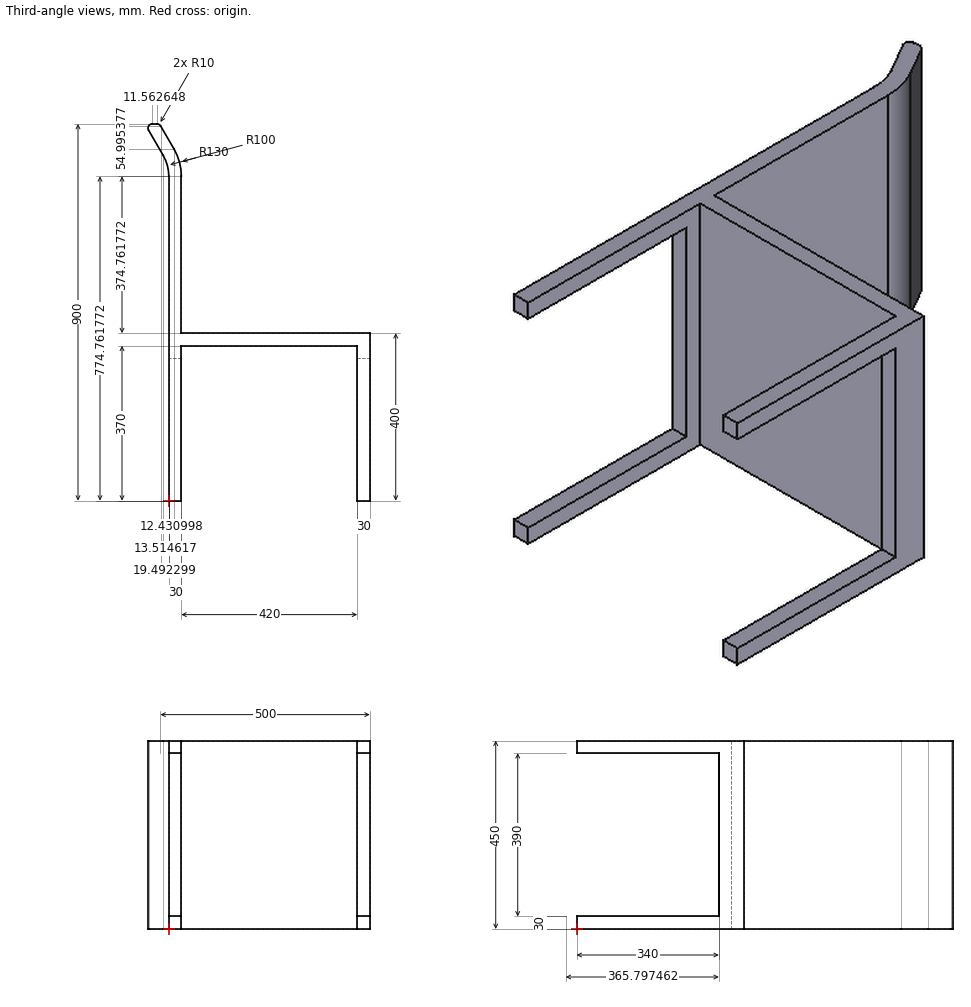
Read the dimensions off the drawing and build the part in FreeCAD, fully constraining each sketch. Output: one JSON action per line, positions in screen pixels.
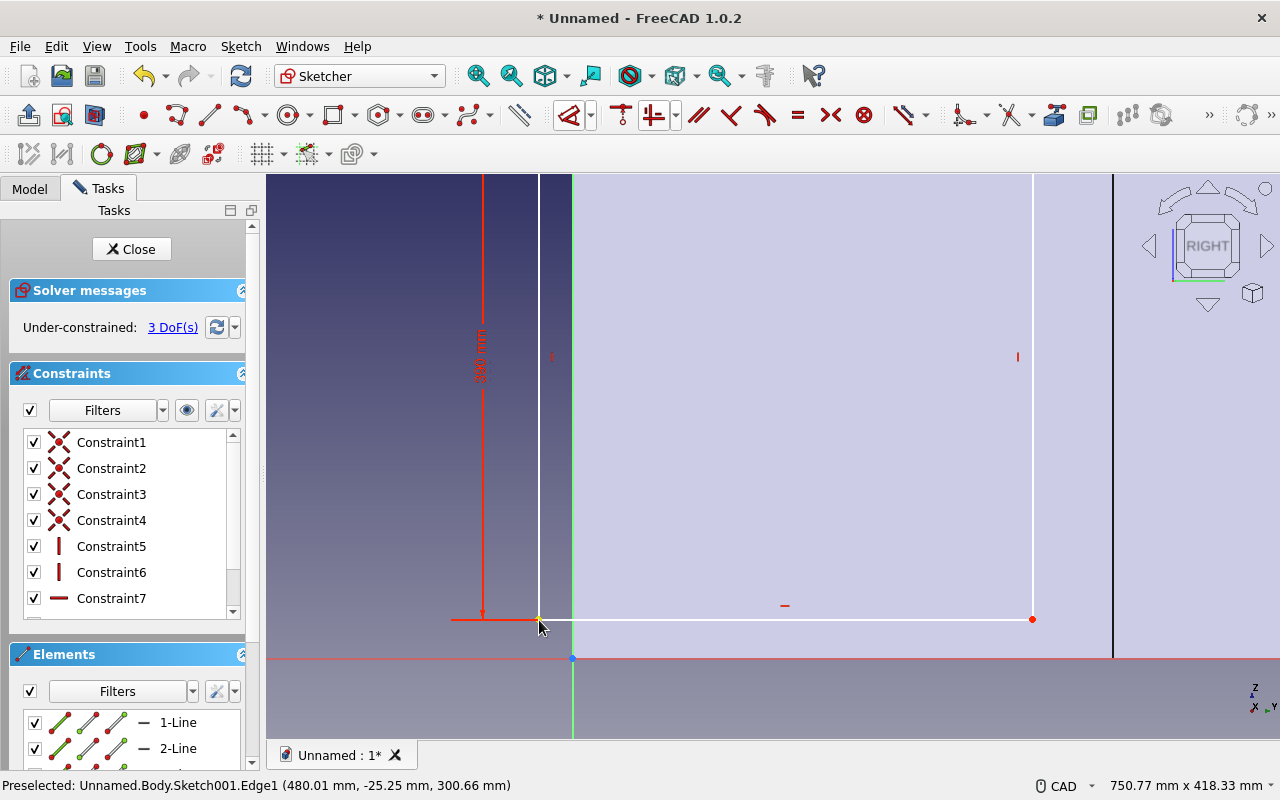
{"action": "left_click", "coordinate": [539, 620]}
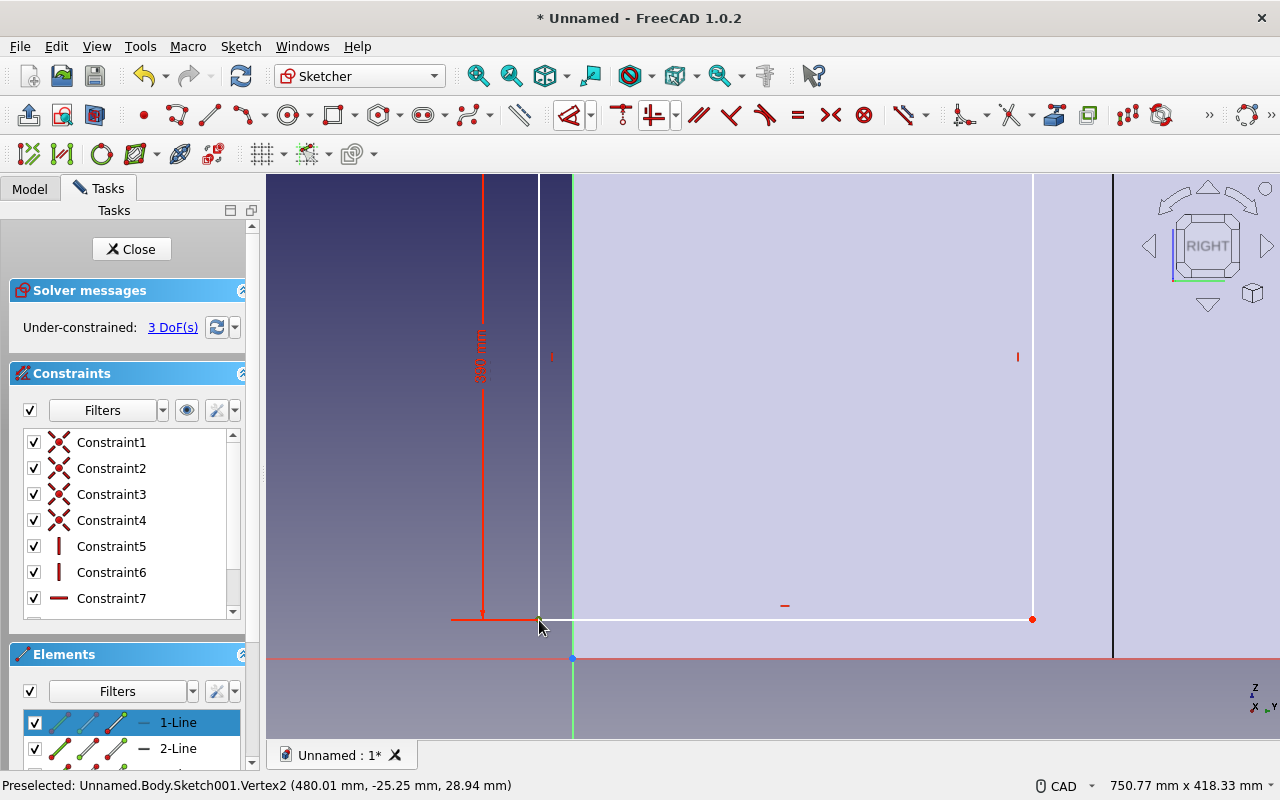
{"action": "left_click", "coordinate": [590, 116]}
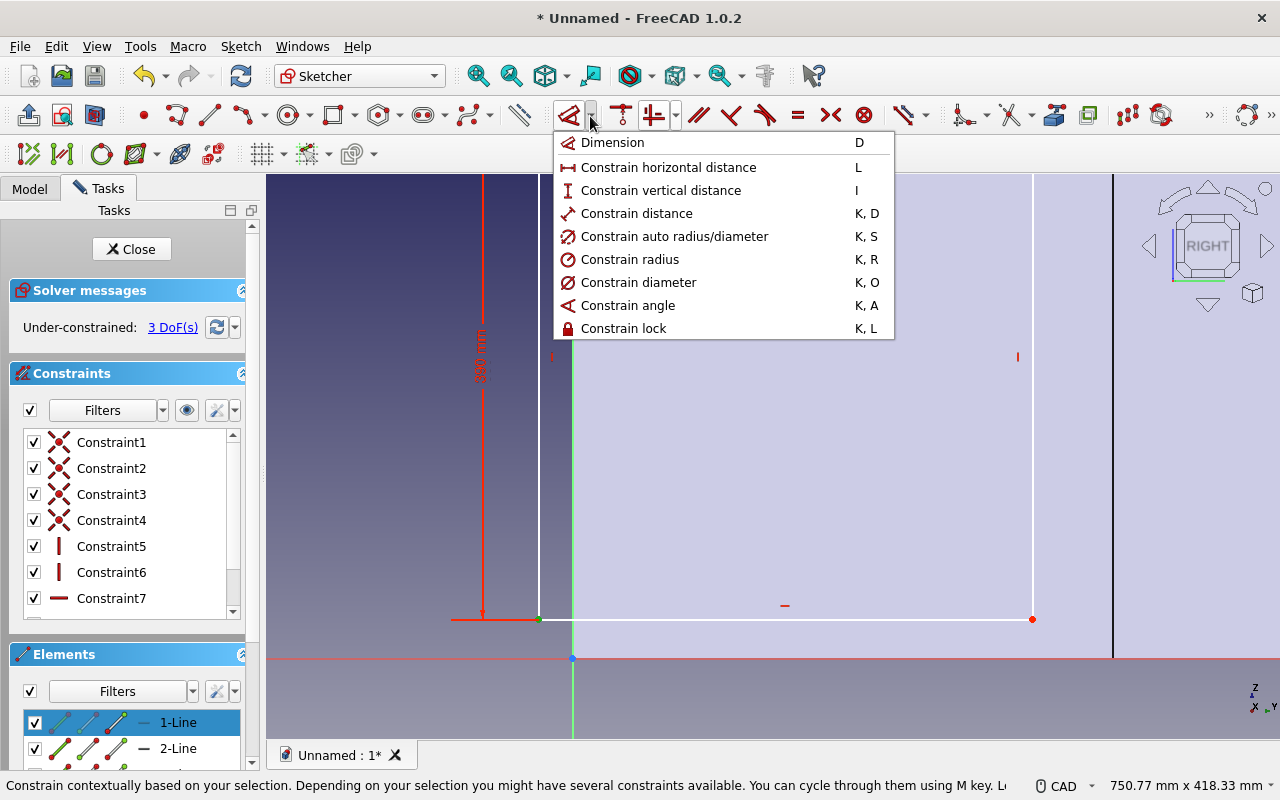
{"action": "left_click", "coordinate": [724, 190]}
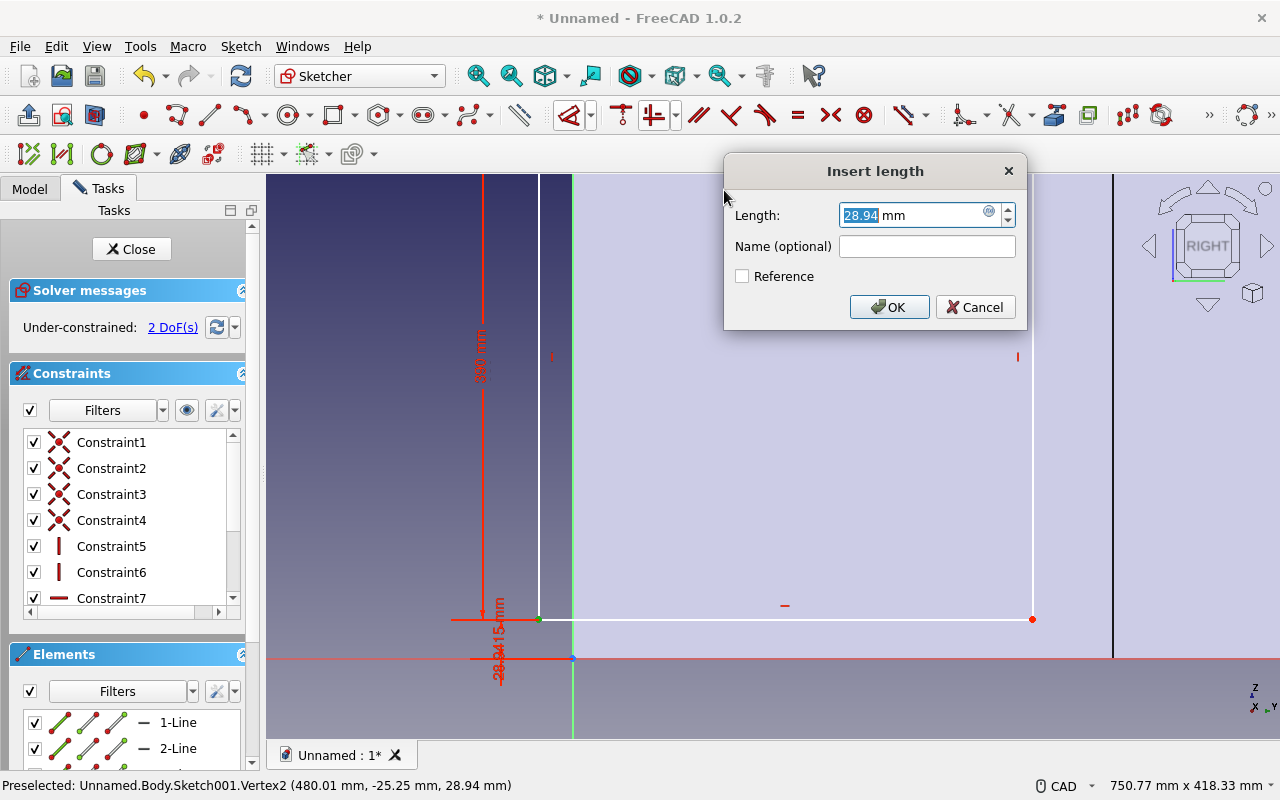
{"action": "type", "text": "30"}
{"action": "key", "text": "Return"}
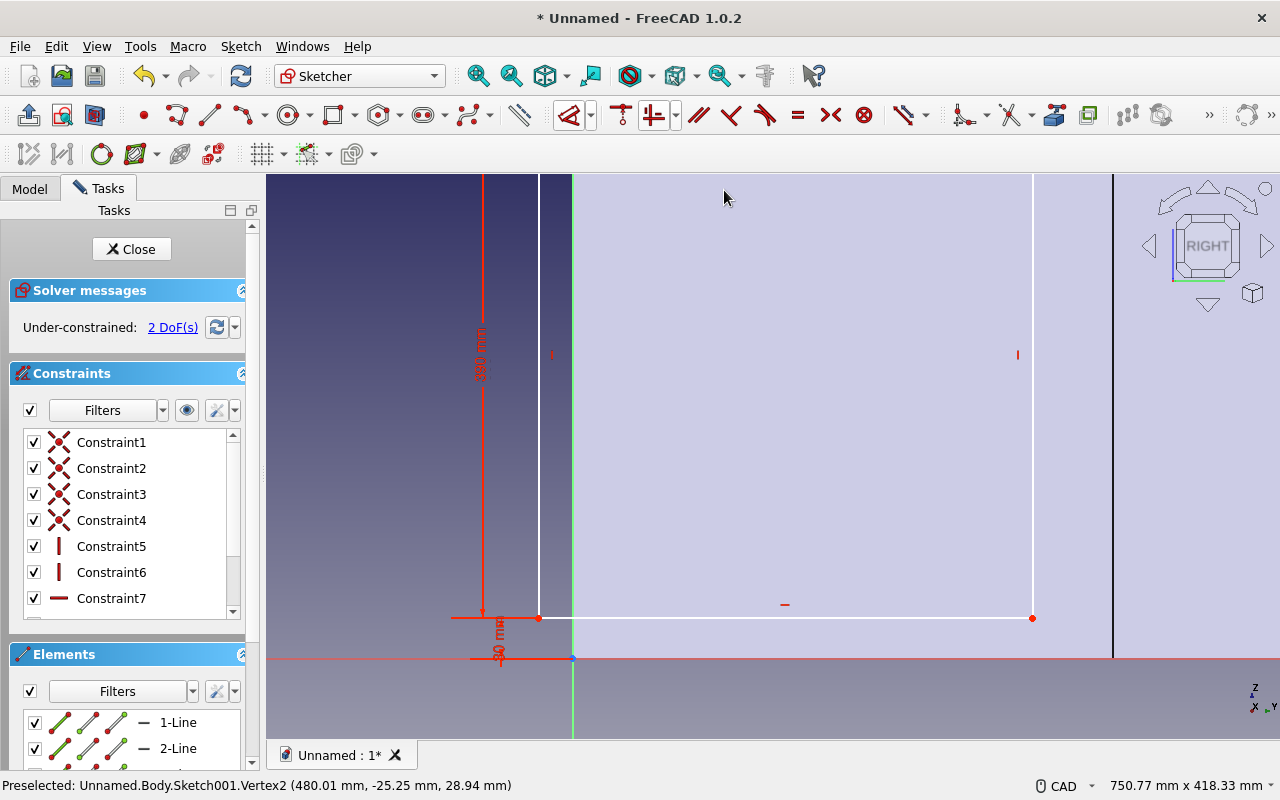
{"action": "left_click", "coordinate": [1033, 618]}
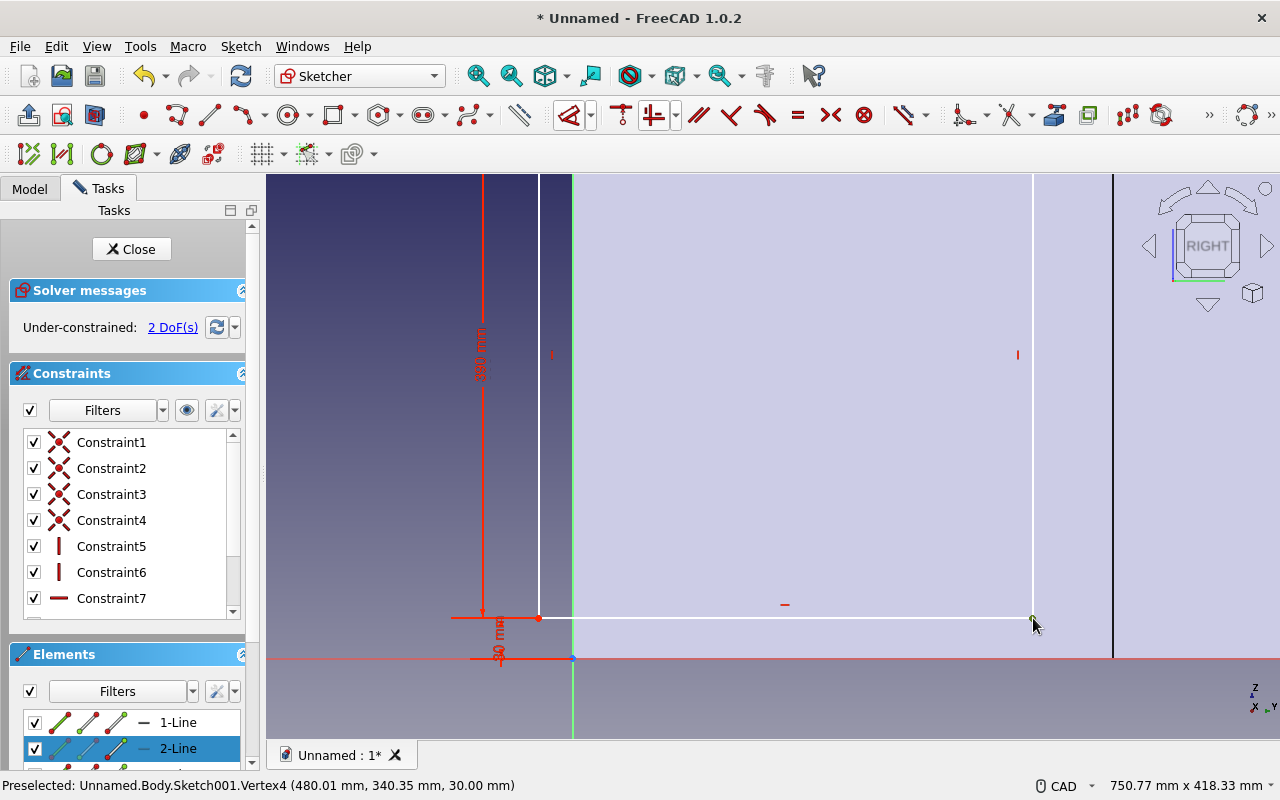
{"action": "left_click", "coordinate": [590, 116]}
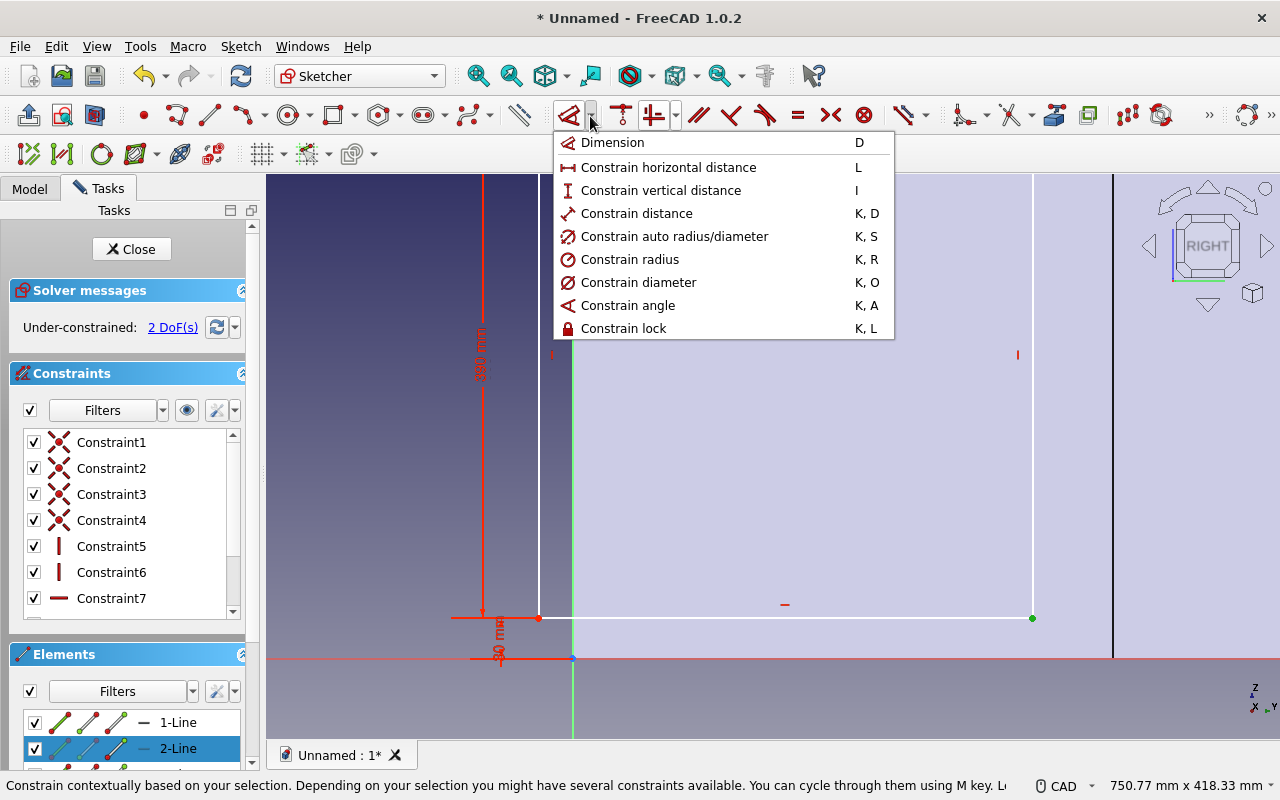
{"action": "left_click", "coordinate": [724, 168]}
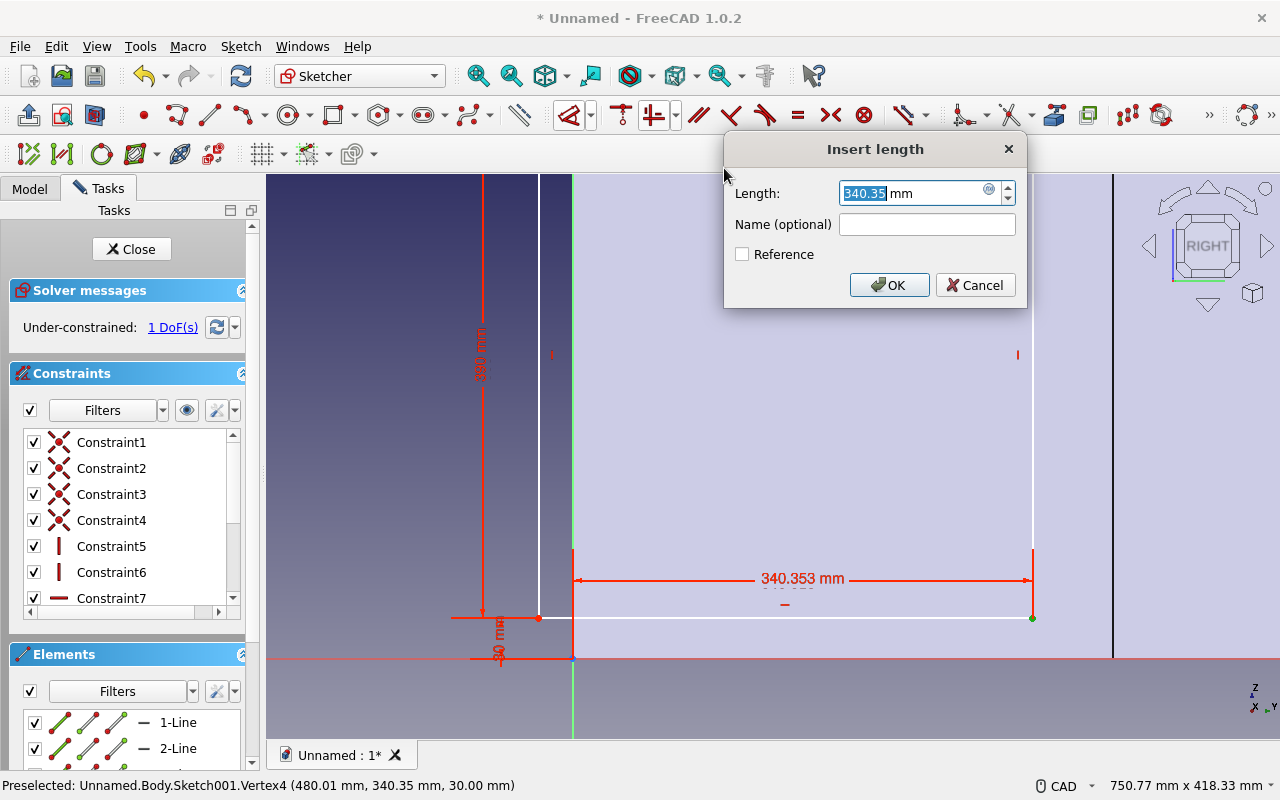
{"action": "type", "text": "340"}
{"action": "key", "text": "Return"}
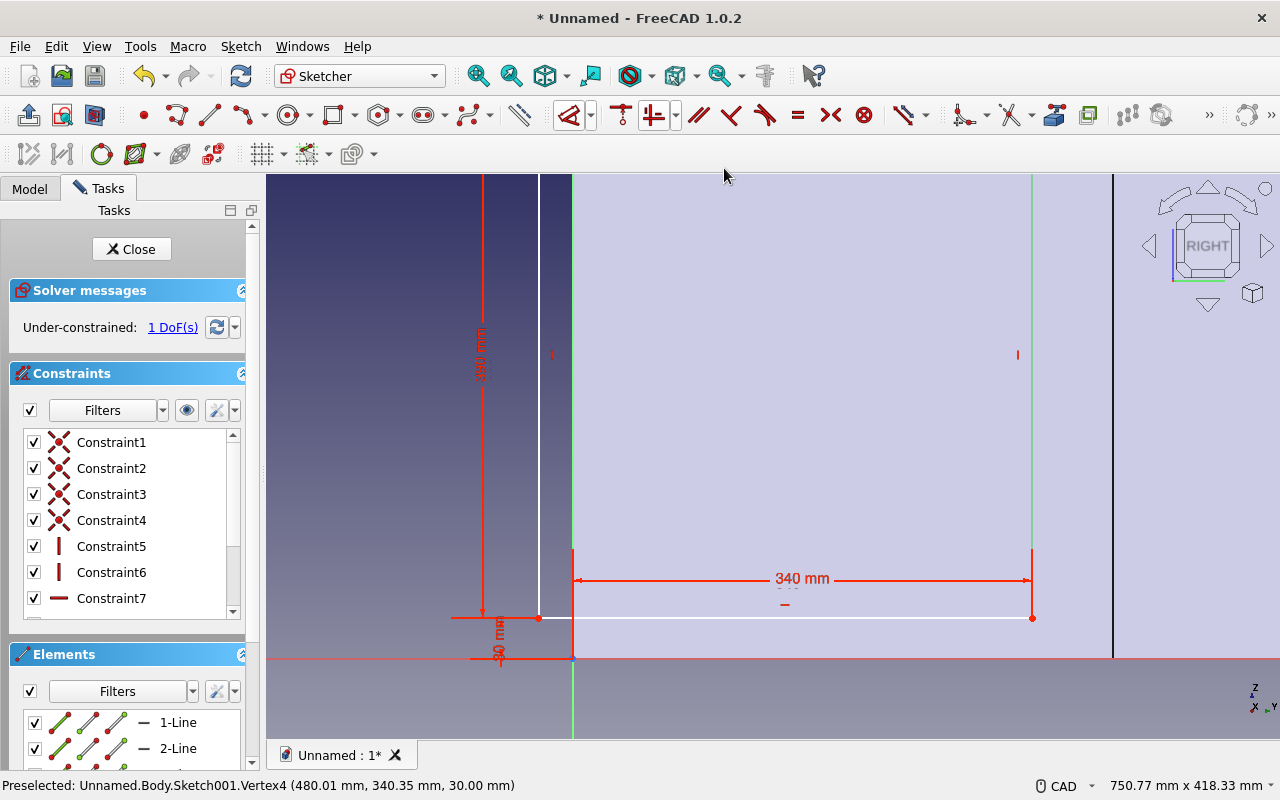
{"action": "left_click", "coordinate": [687, 618]}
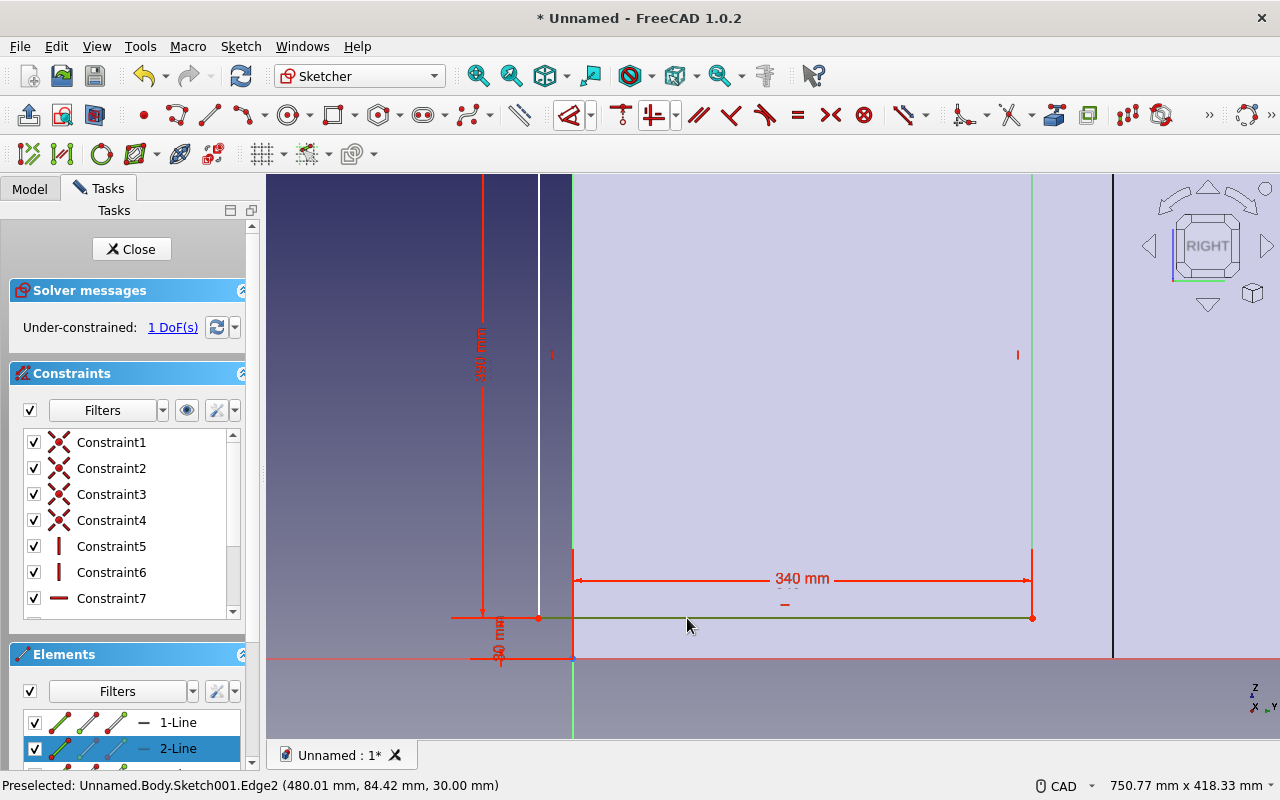
{"action": "left_click", "coordinate": [590, 116]}